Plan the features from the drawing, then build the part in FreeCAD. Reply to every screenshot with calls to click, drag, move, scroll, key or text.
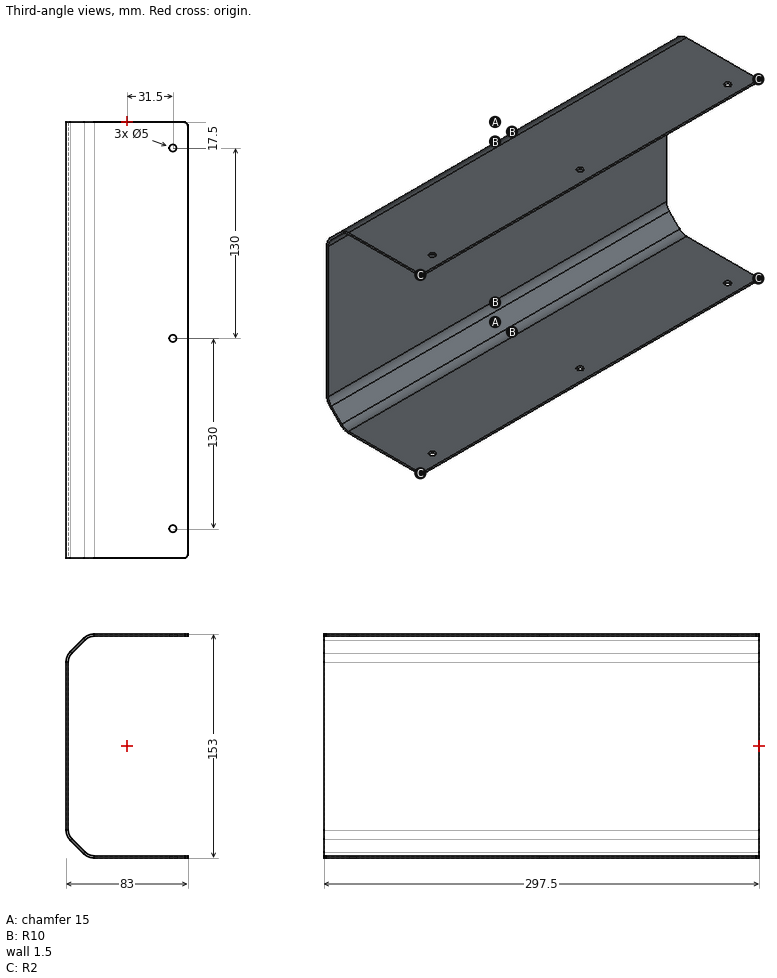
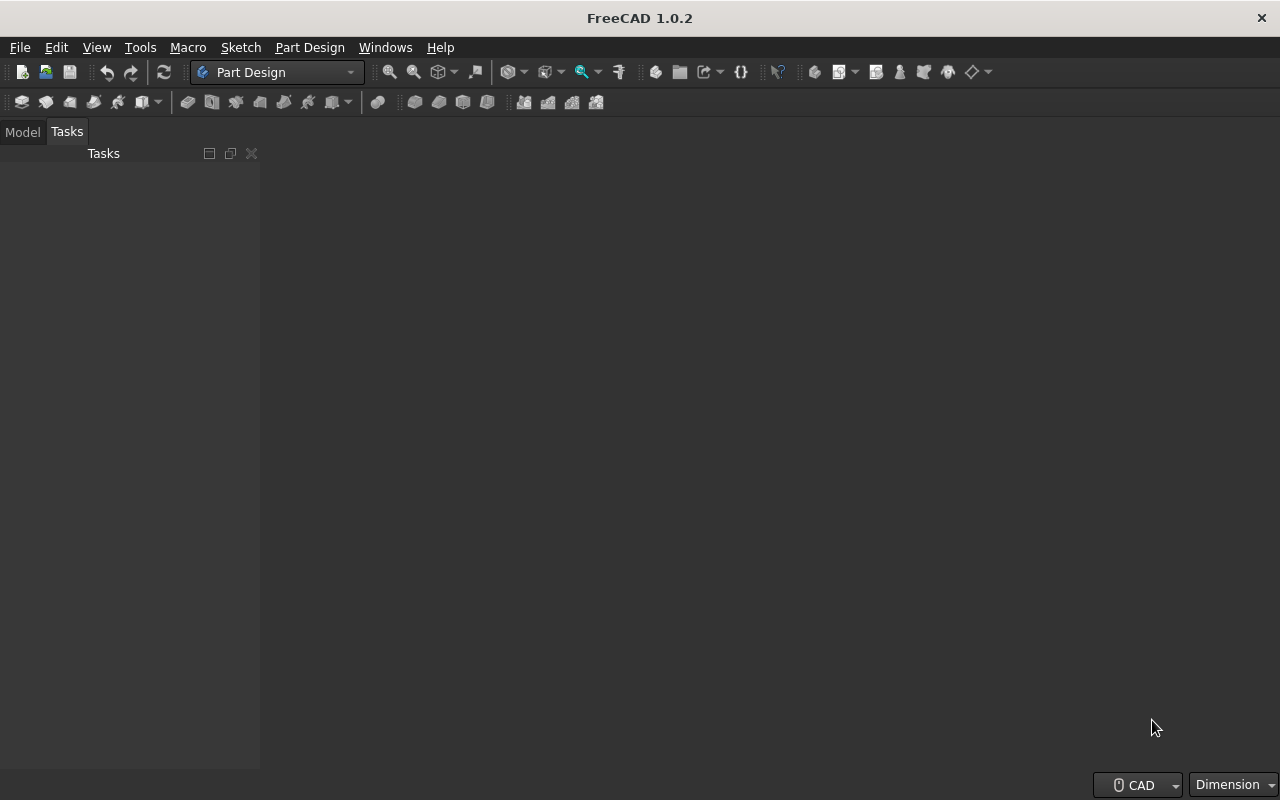
click(22, 72)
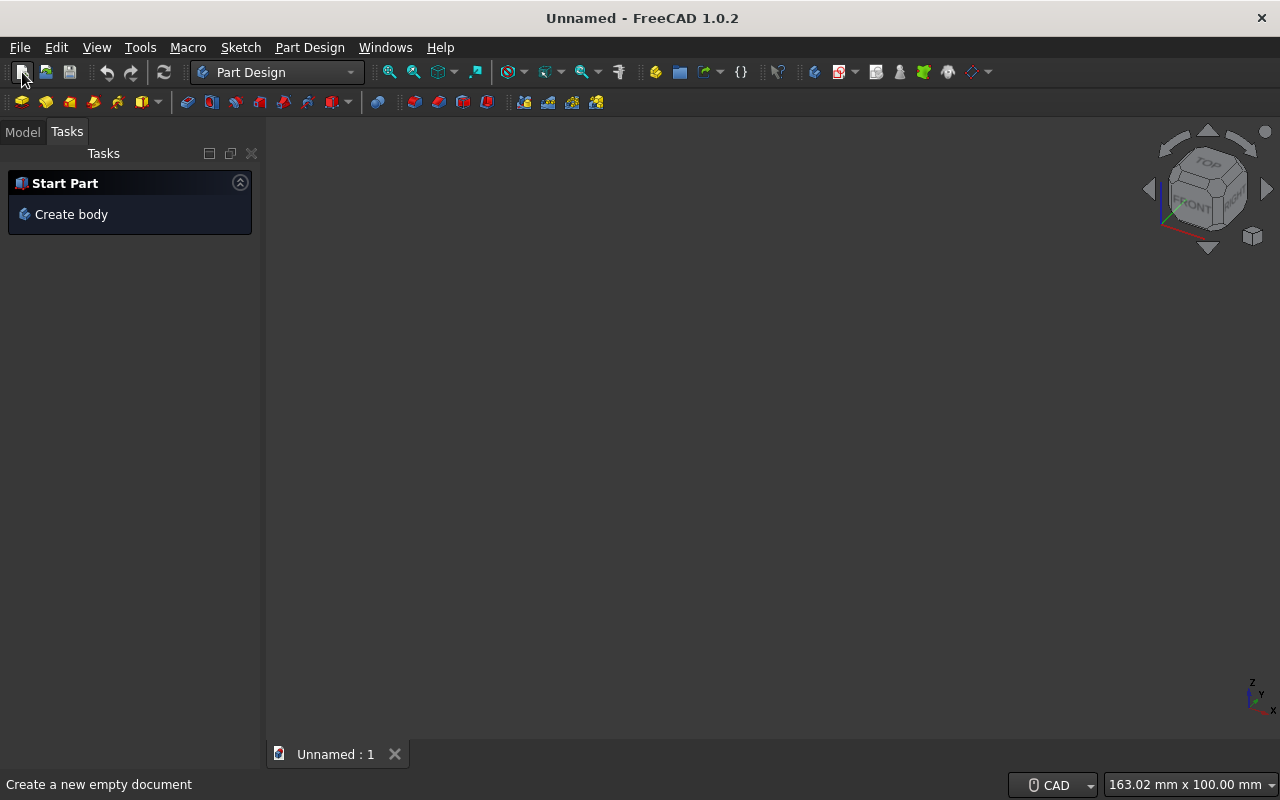
click(840, 72)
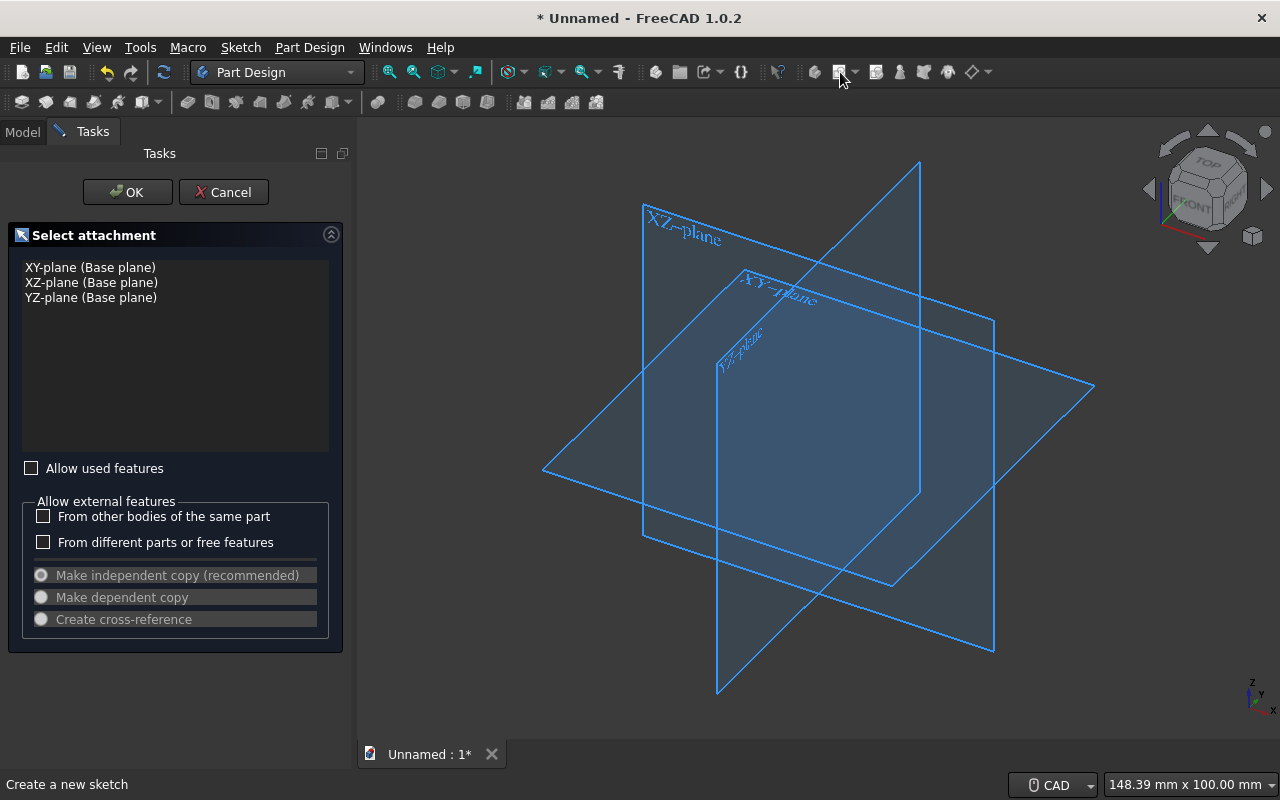
click(82, 282)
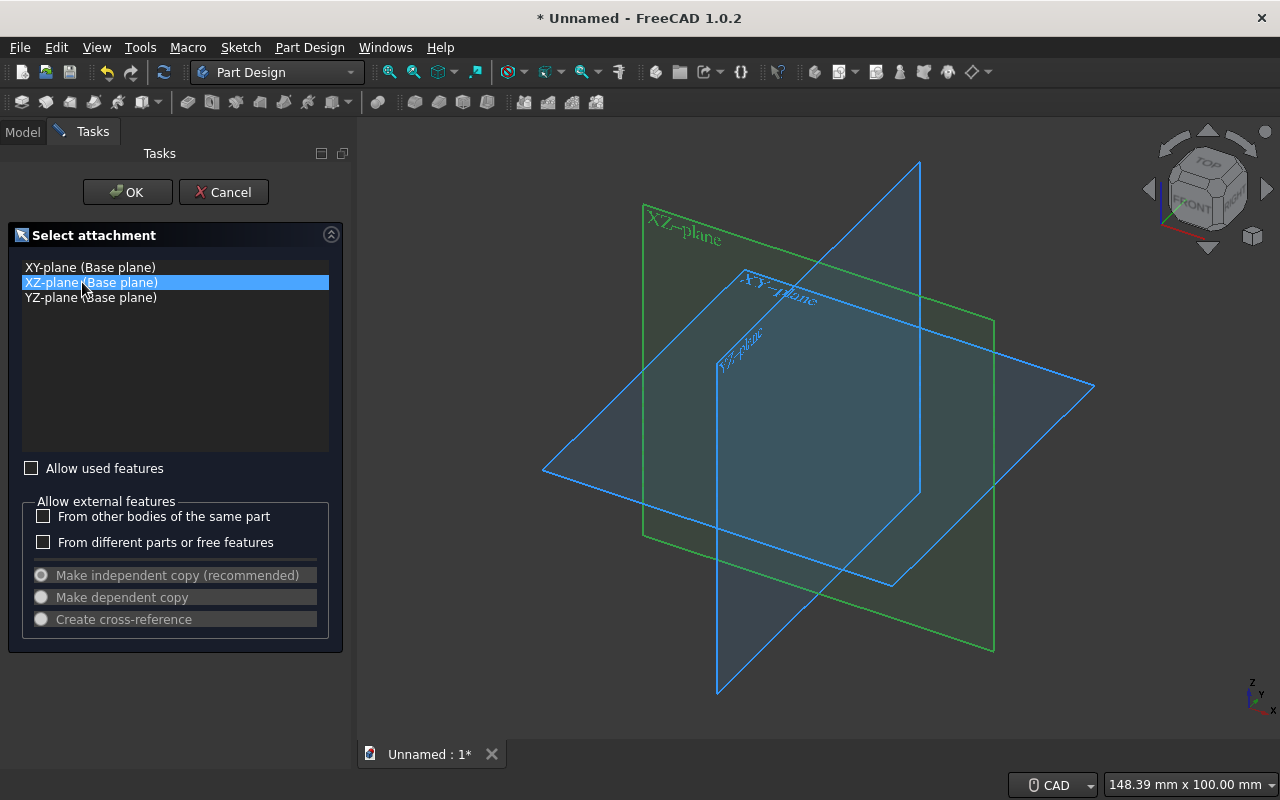
click(128, 192)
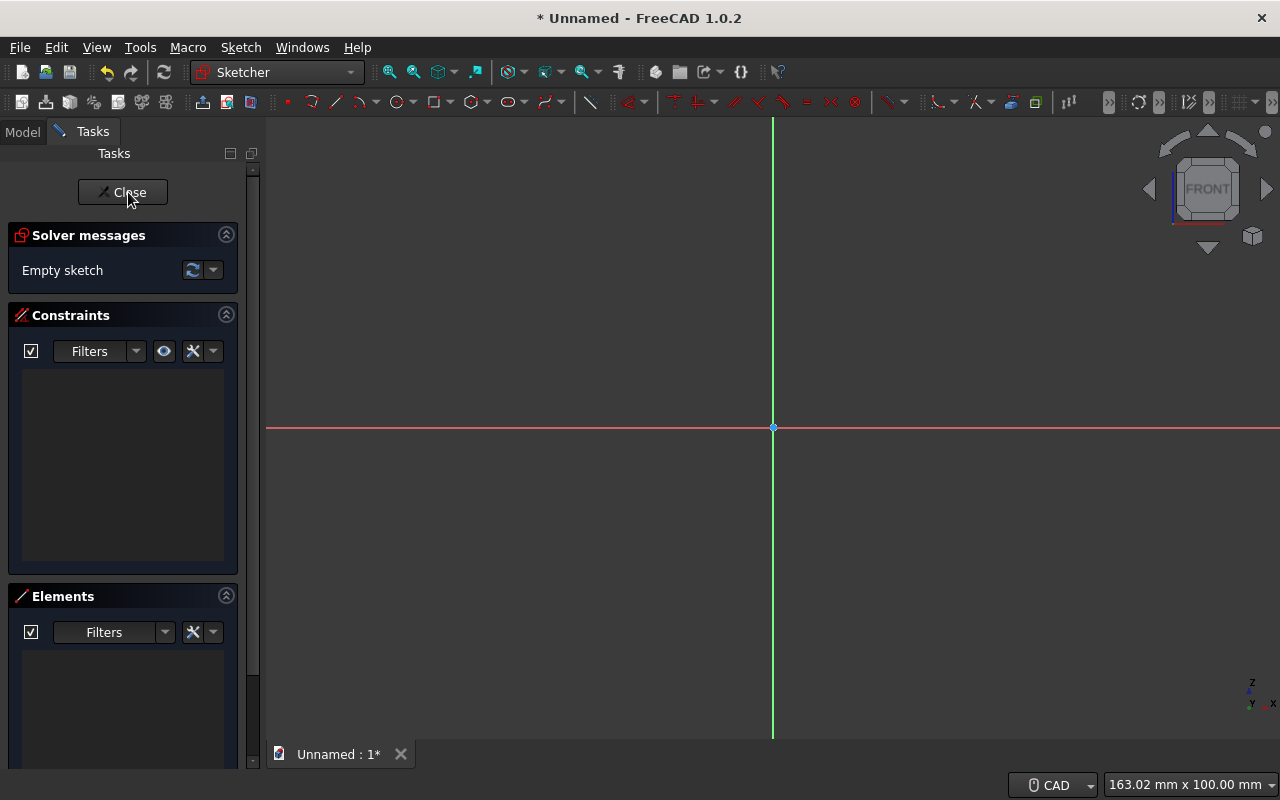
scroll(649, 428, down, 4)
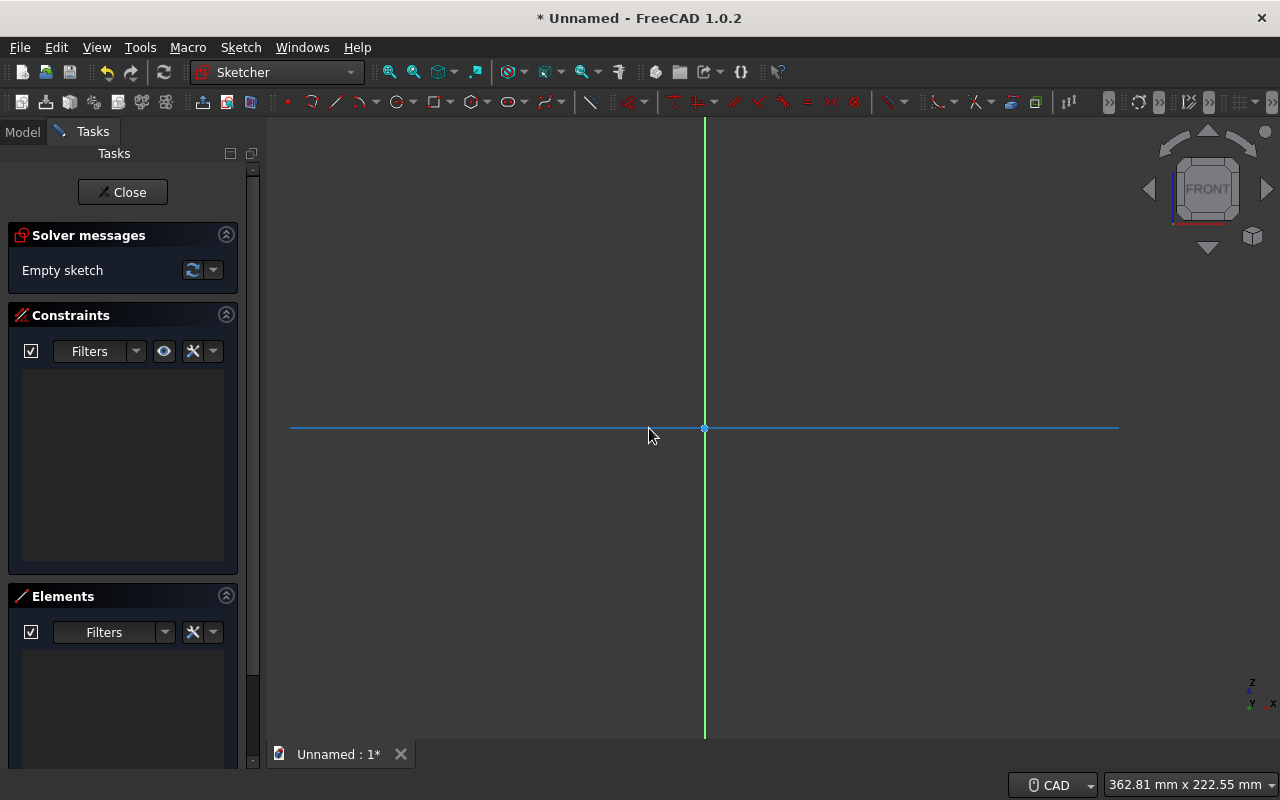
key(g)
key(v)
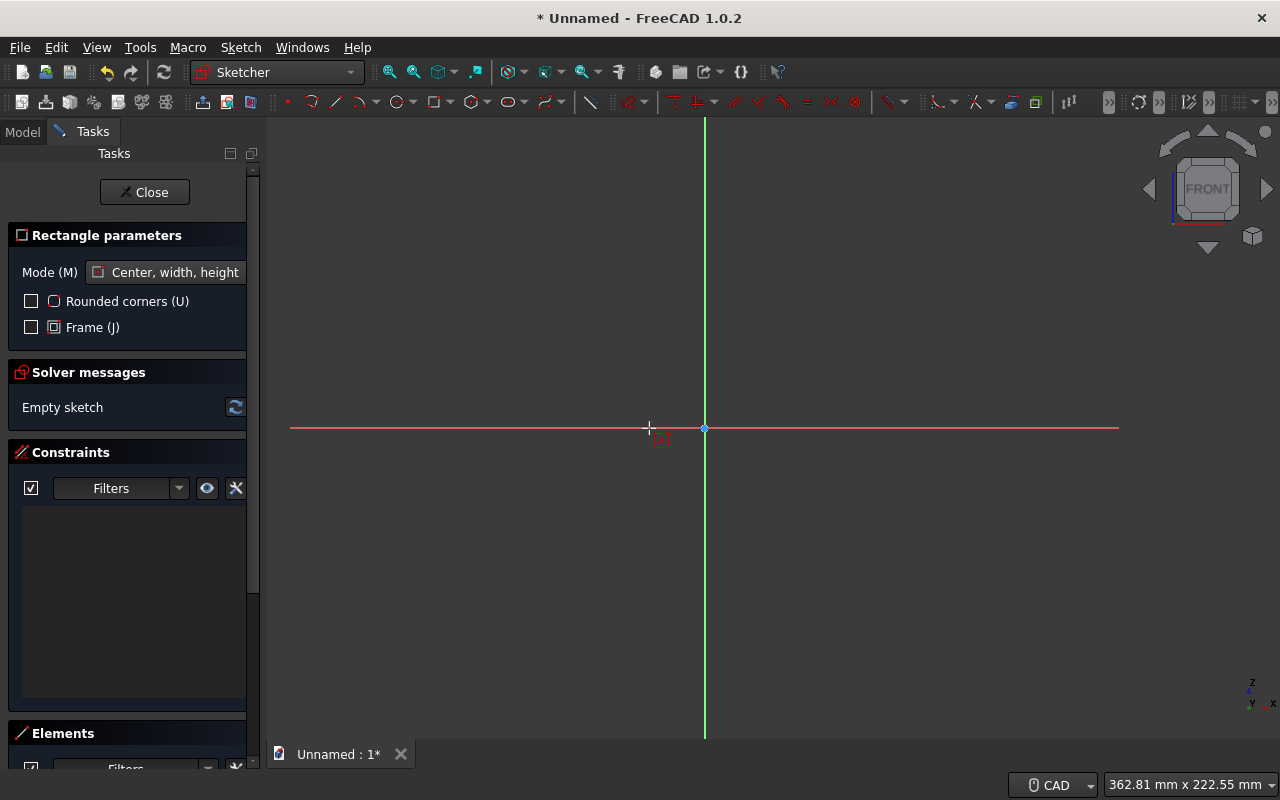
click(705, 428)
click(821, 214)
key(Escape)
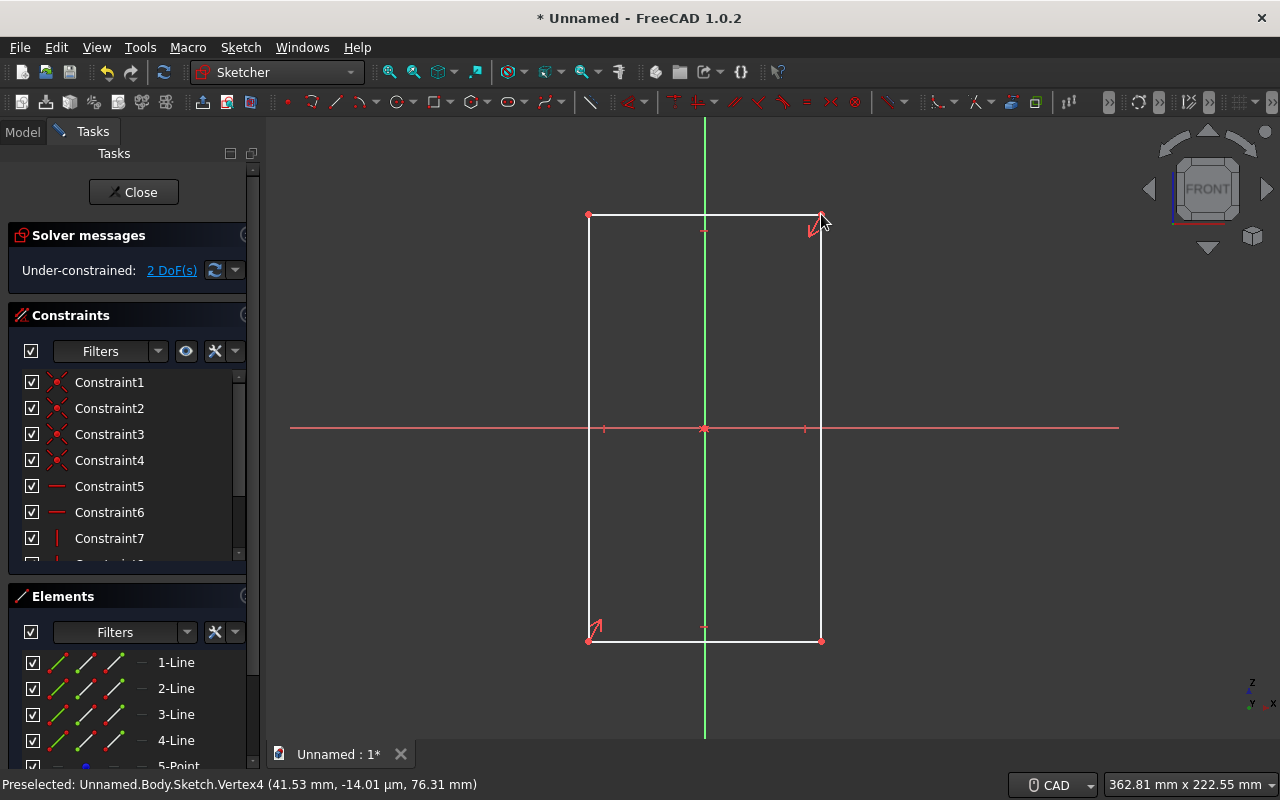
key(d)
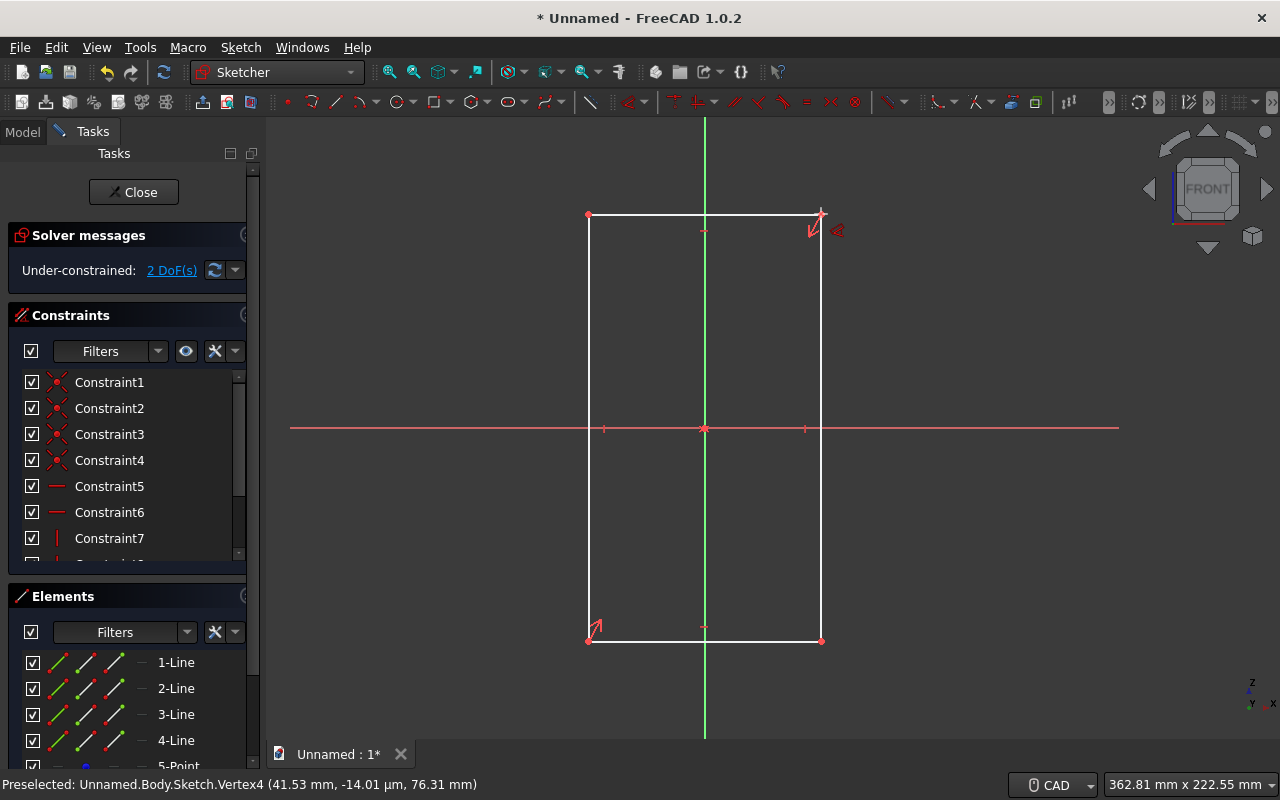
click(658, 642)
click(652, 676)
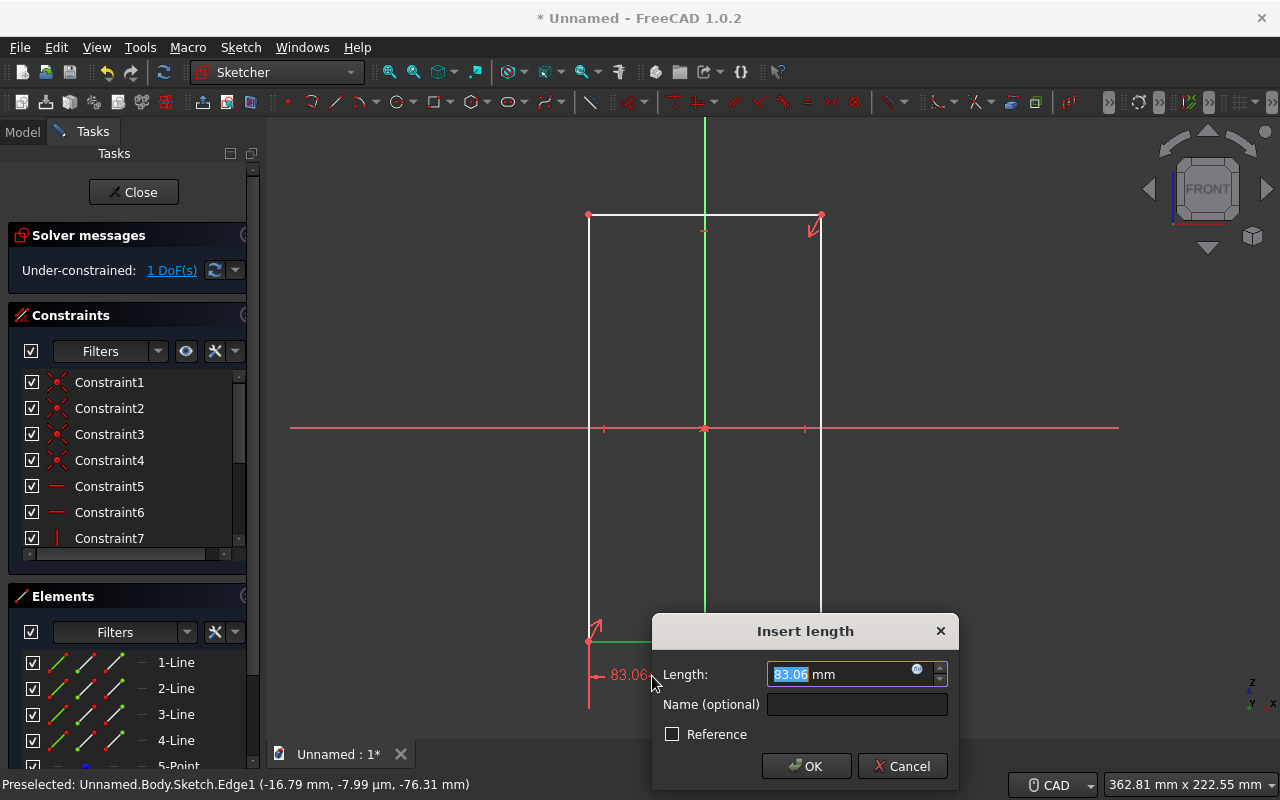
text(83)
key(Return)